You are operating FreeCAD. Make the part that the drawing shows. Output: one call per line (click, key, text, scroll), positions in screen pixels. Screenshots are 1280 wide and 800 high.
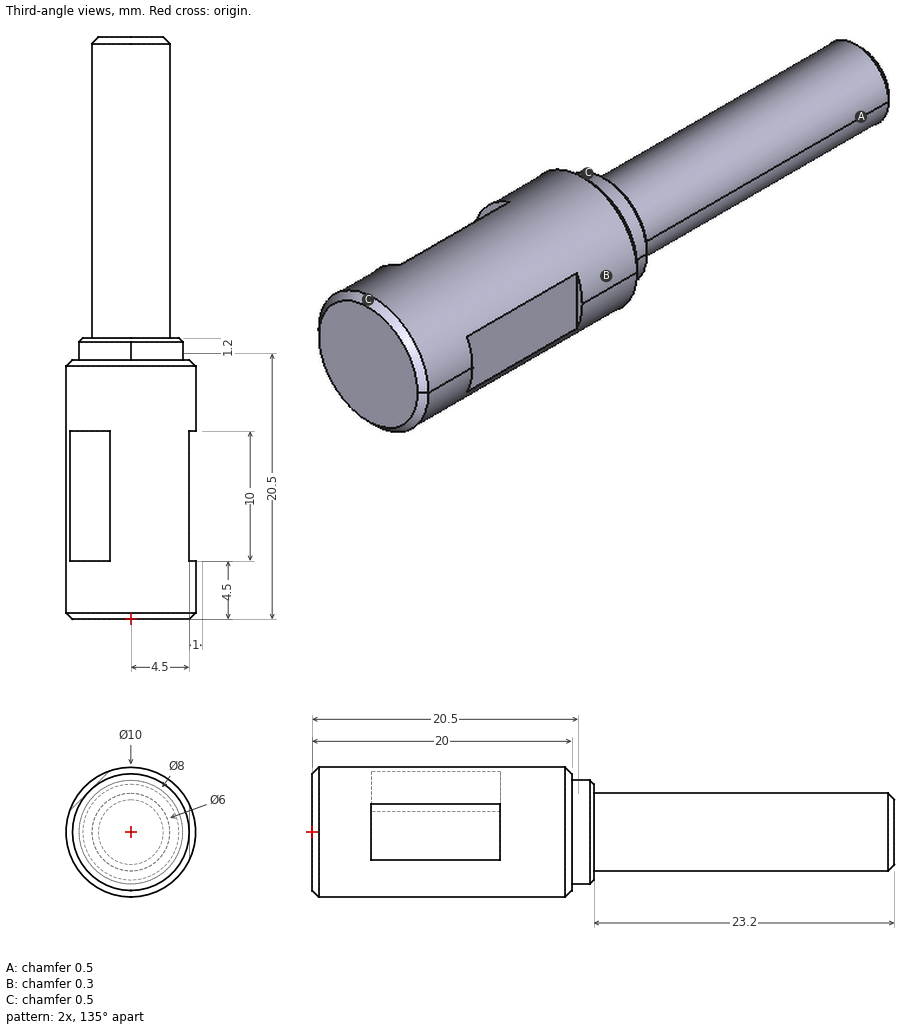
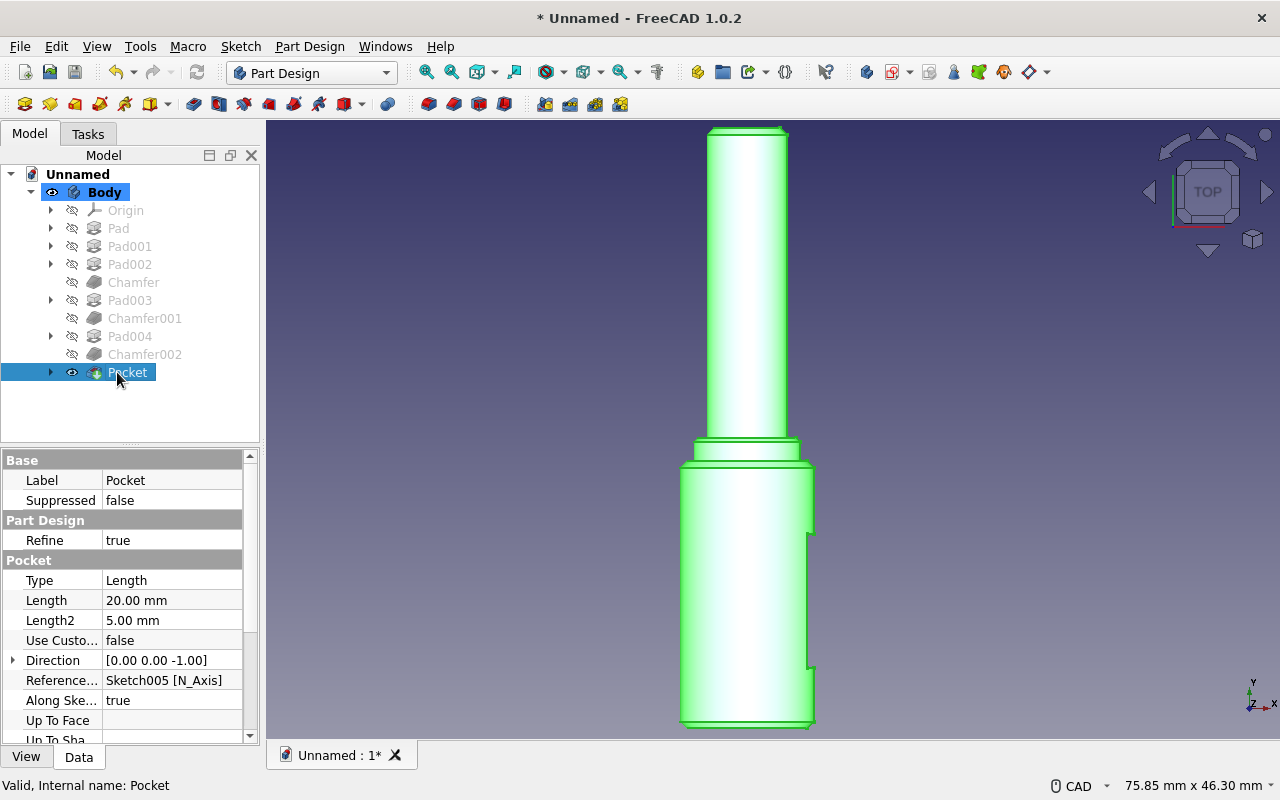
click(595, 104)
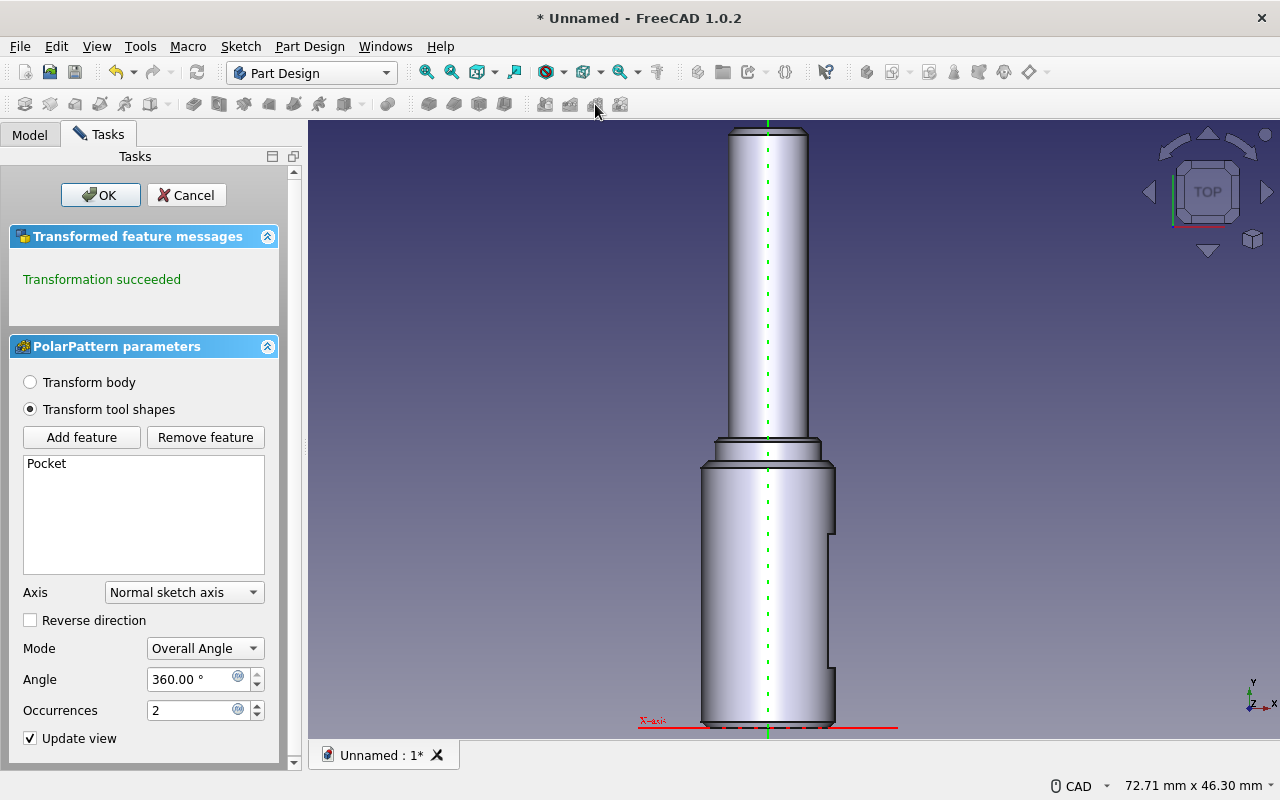
click(185, 592)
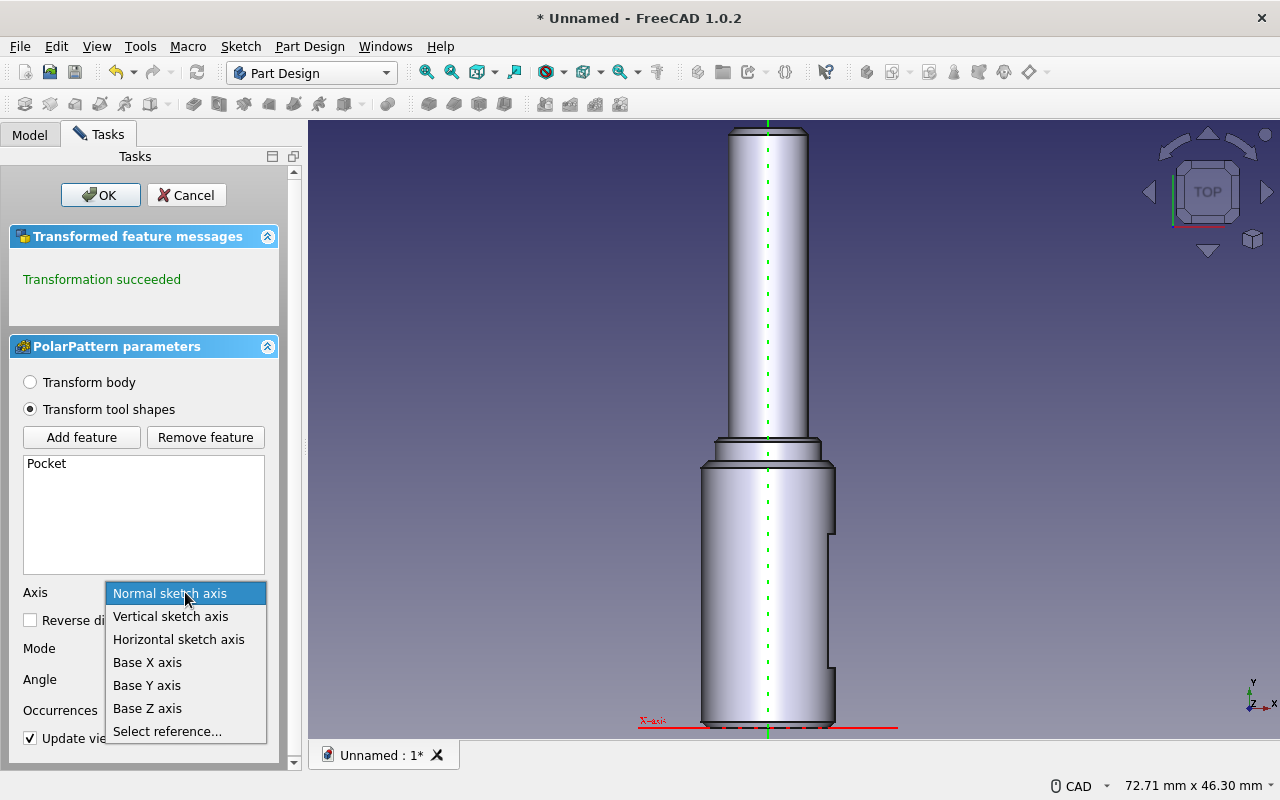
click(184, 686)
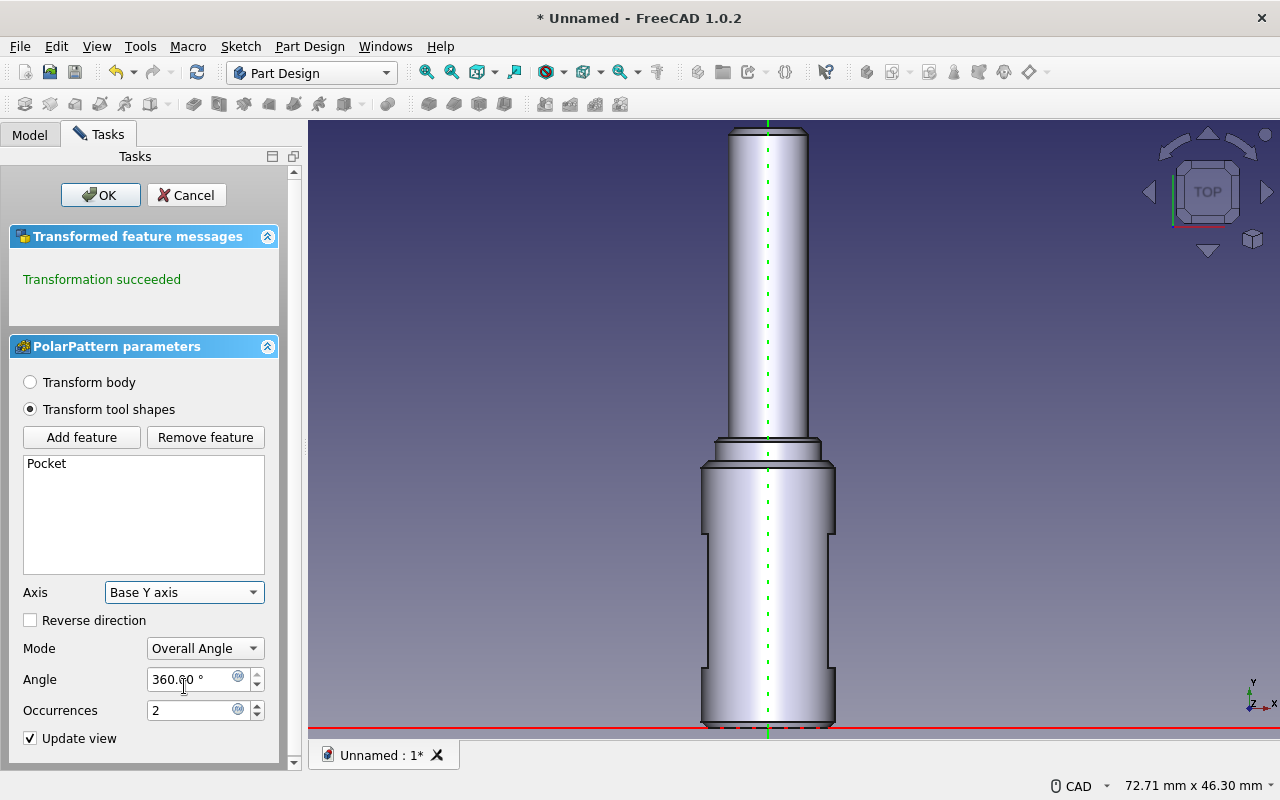
click(206, 648)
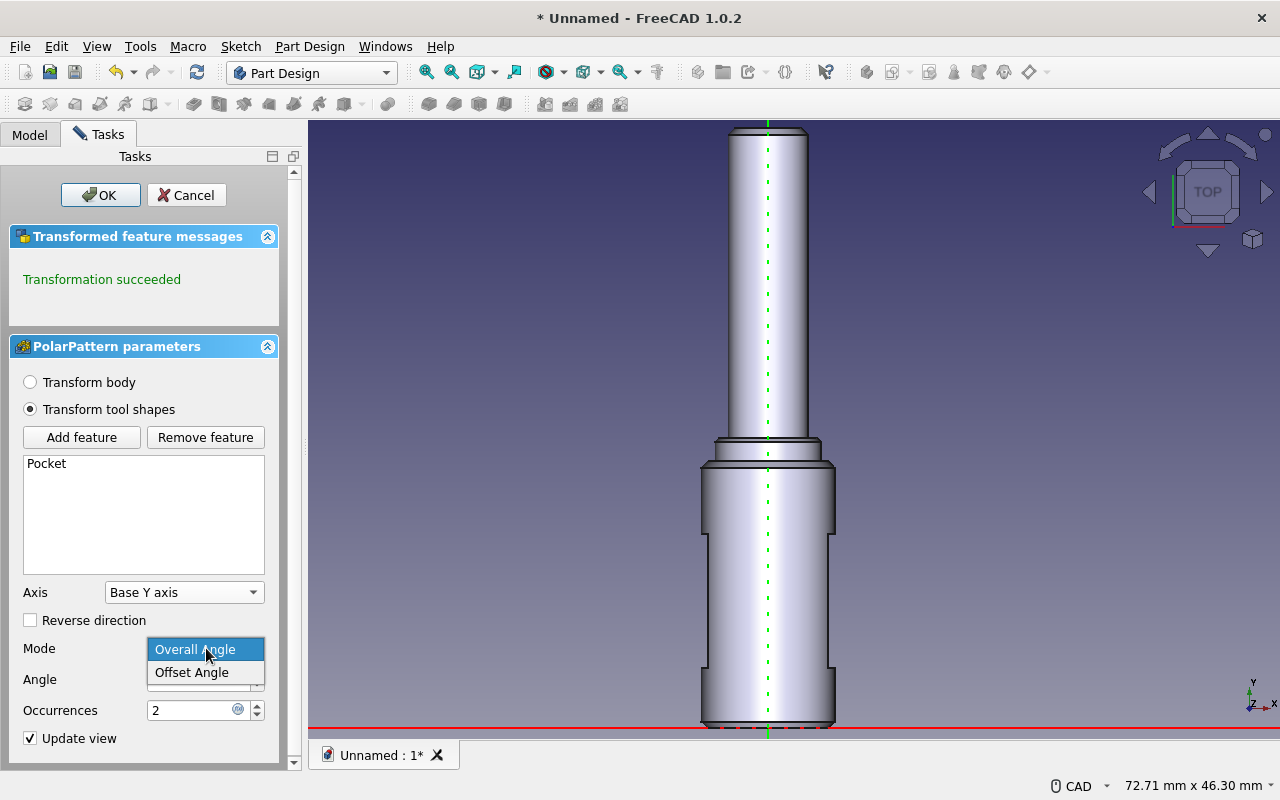
click(204, 672)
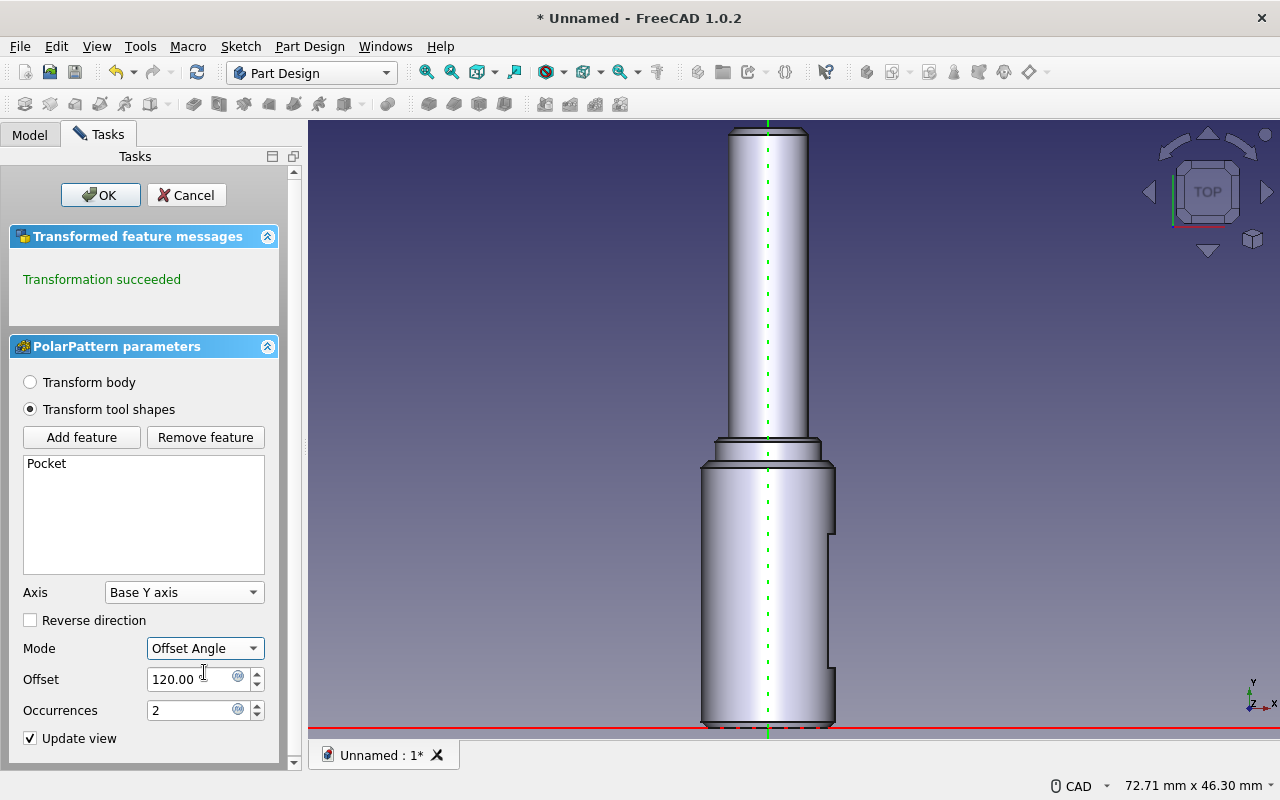
triple_click(199, 680)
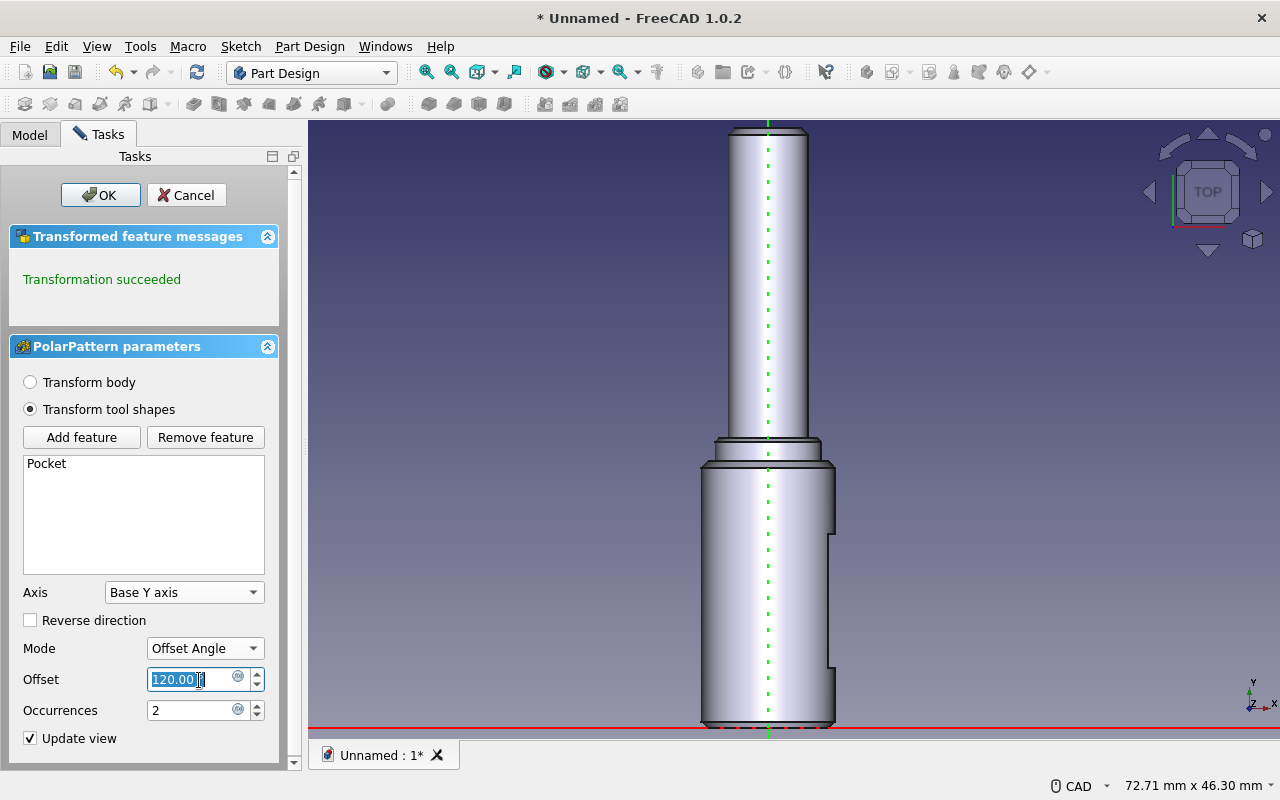
text(135)
key(Tab)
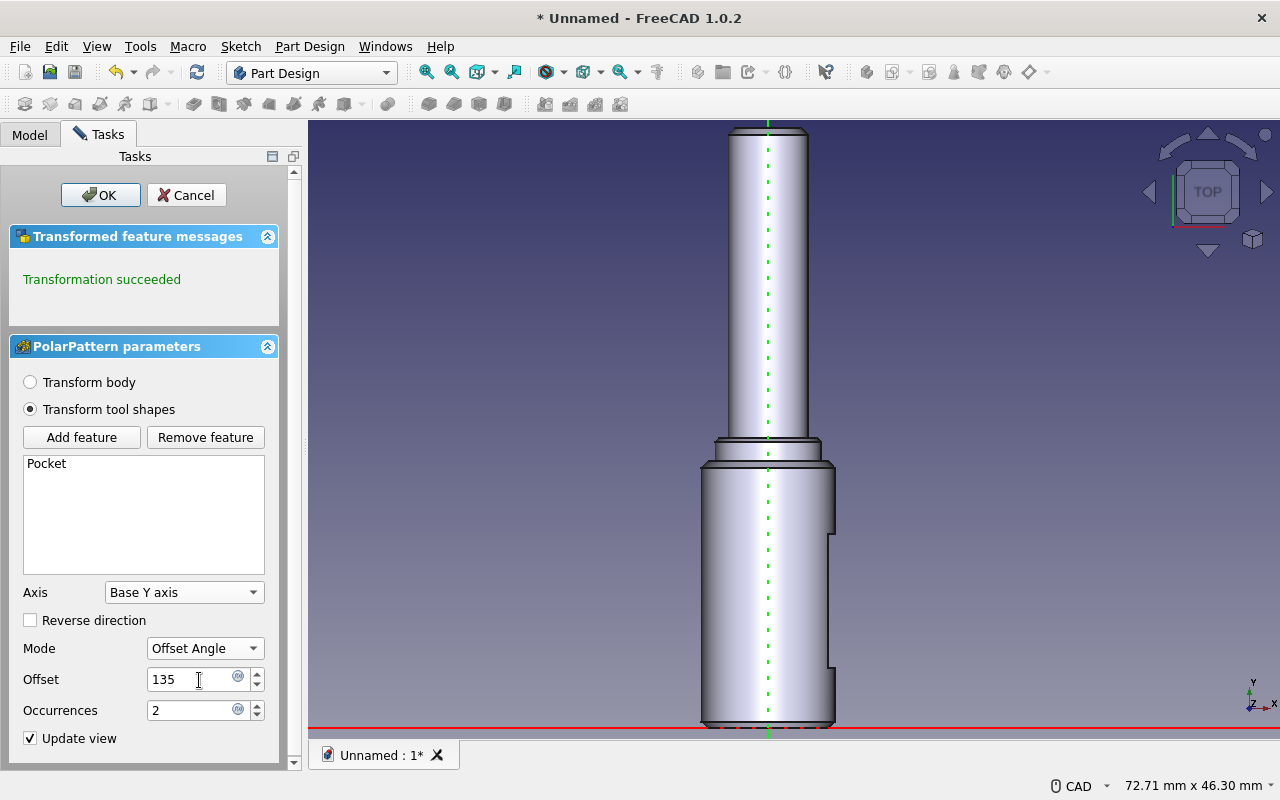
triple_click(199, 710)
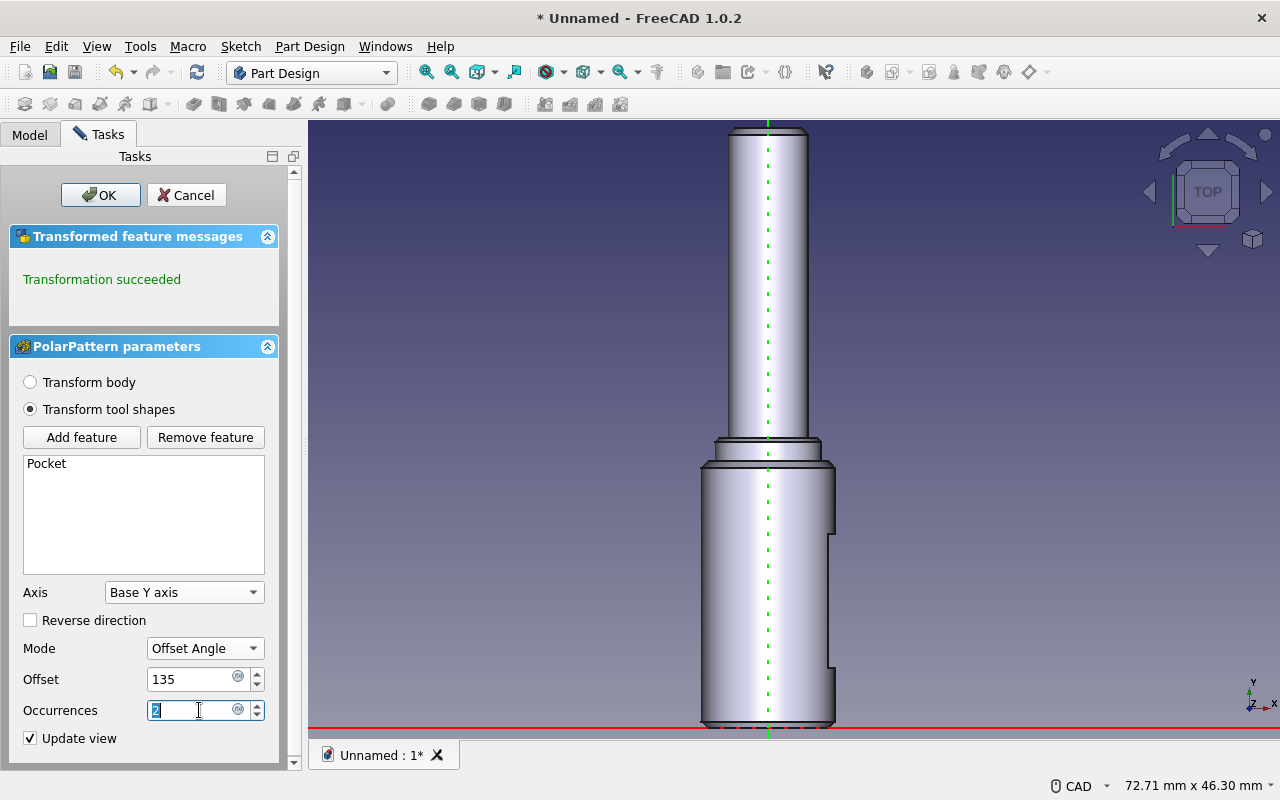
text(2)
key(Tab)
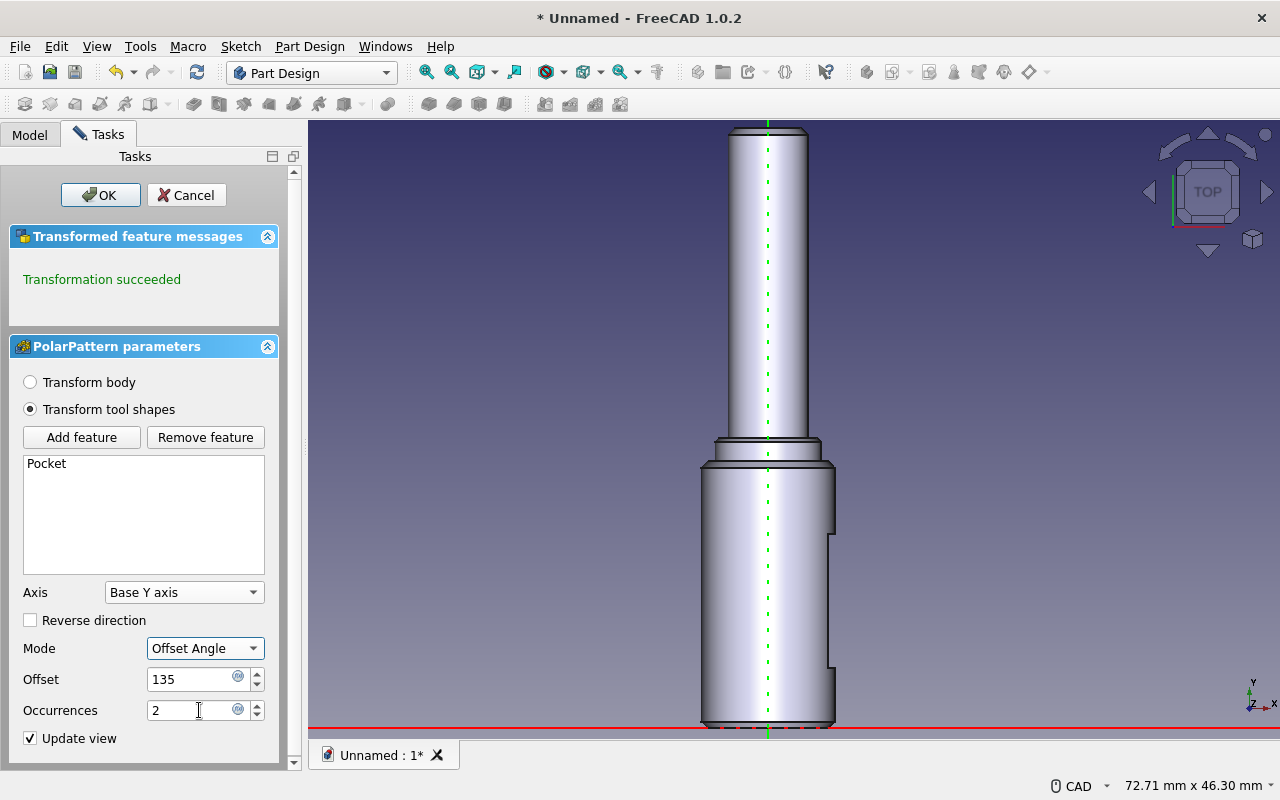
click(31, 620)